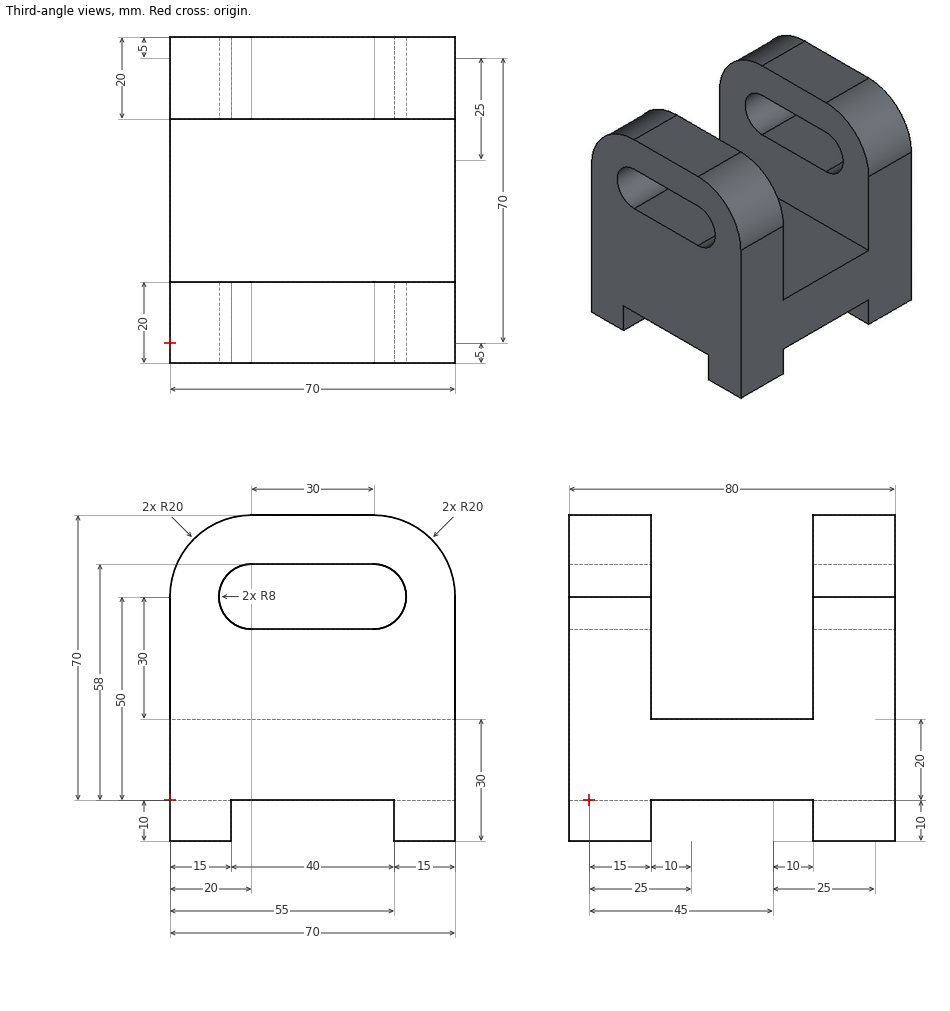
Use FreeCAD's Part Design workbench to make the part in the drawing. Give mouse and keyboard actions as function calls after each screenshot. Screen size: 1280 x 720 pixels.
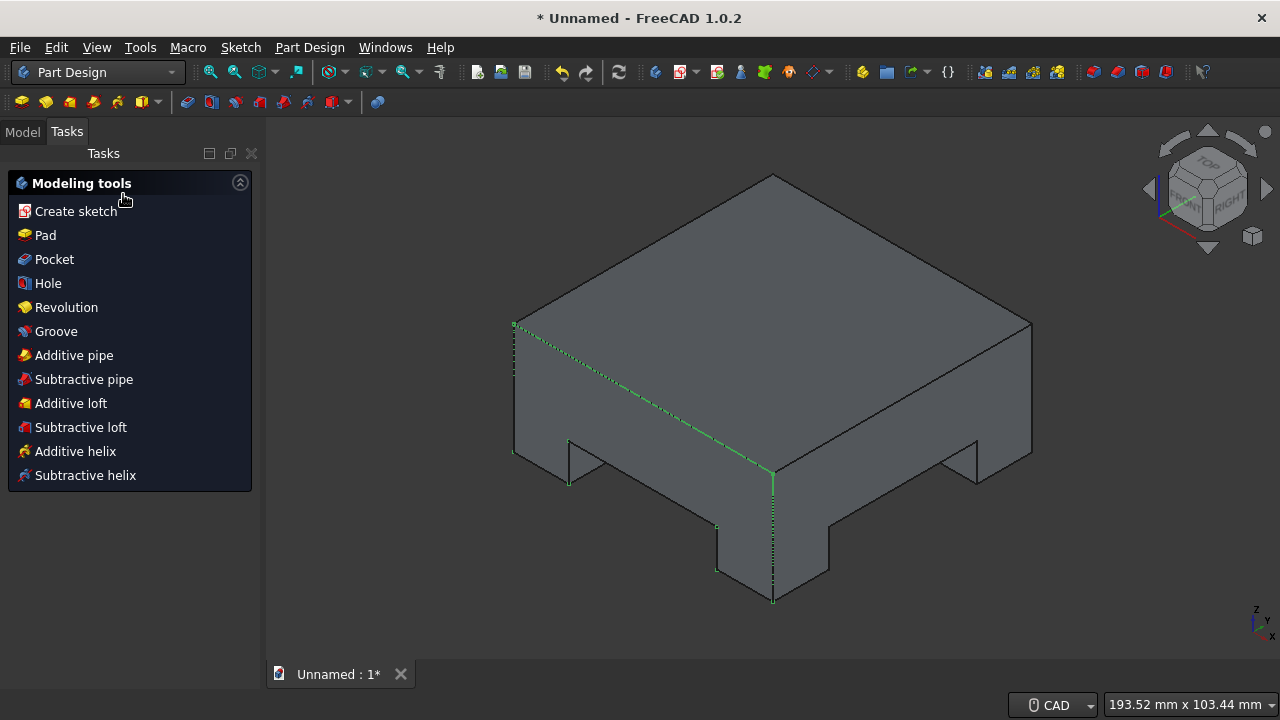
click(22, 102)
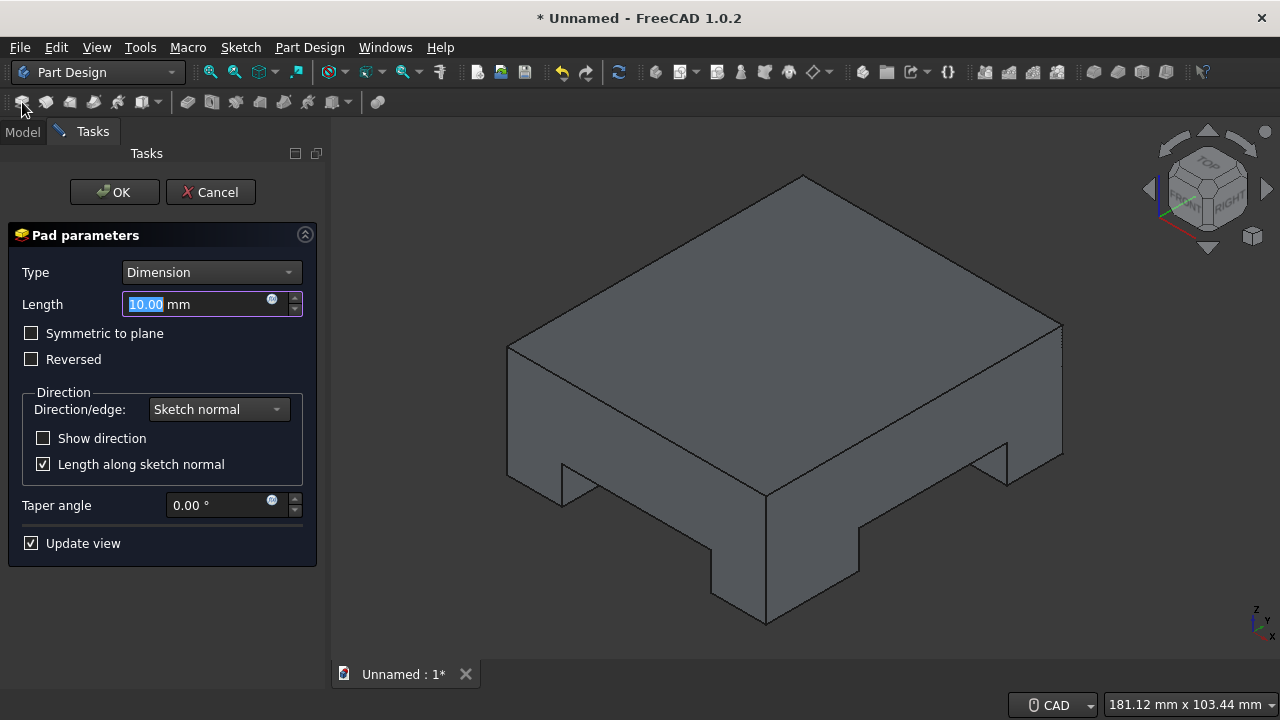
text(5)
key(Tab)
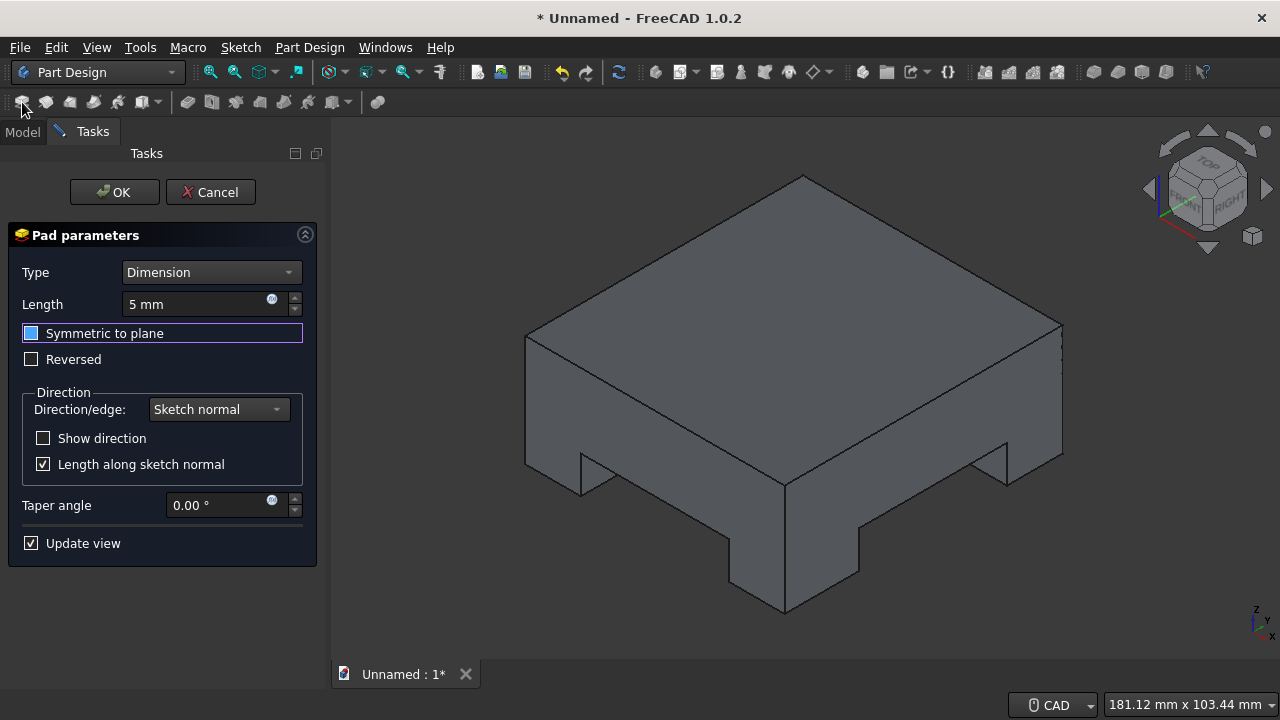
click(115, 192)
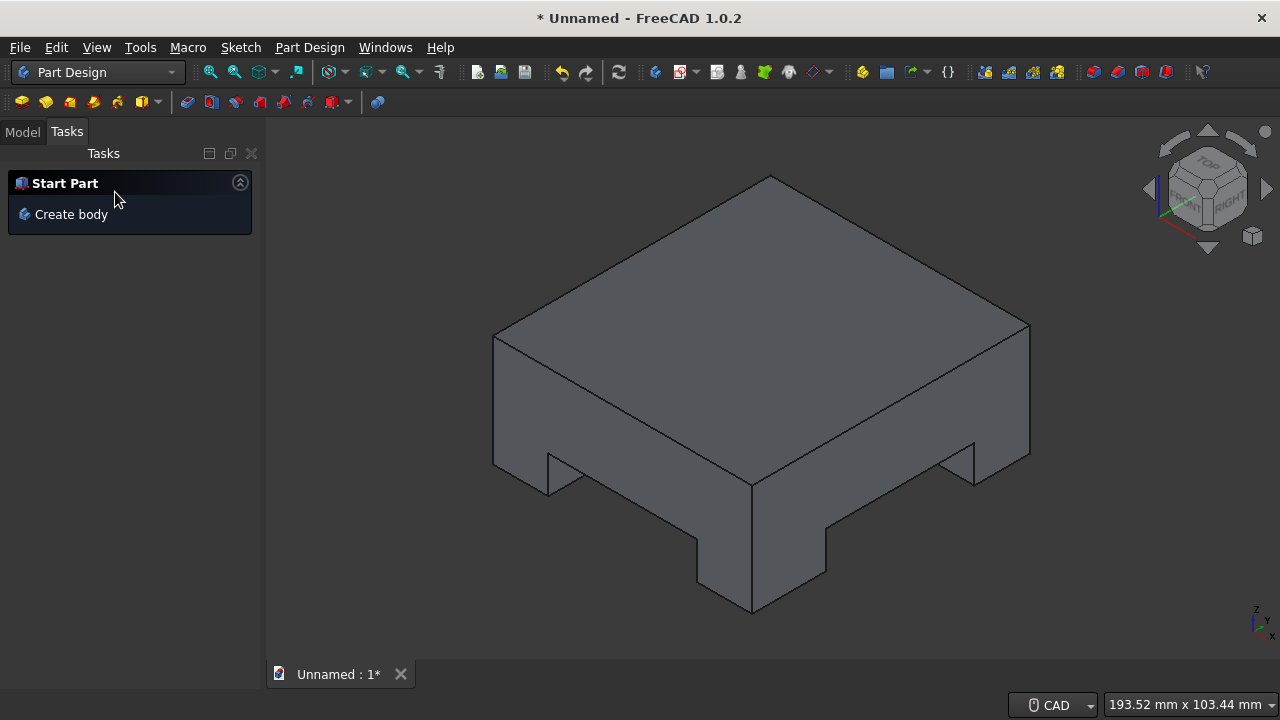
key(4)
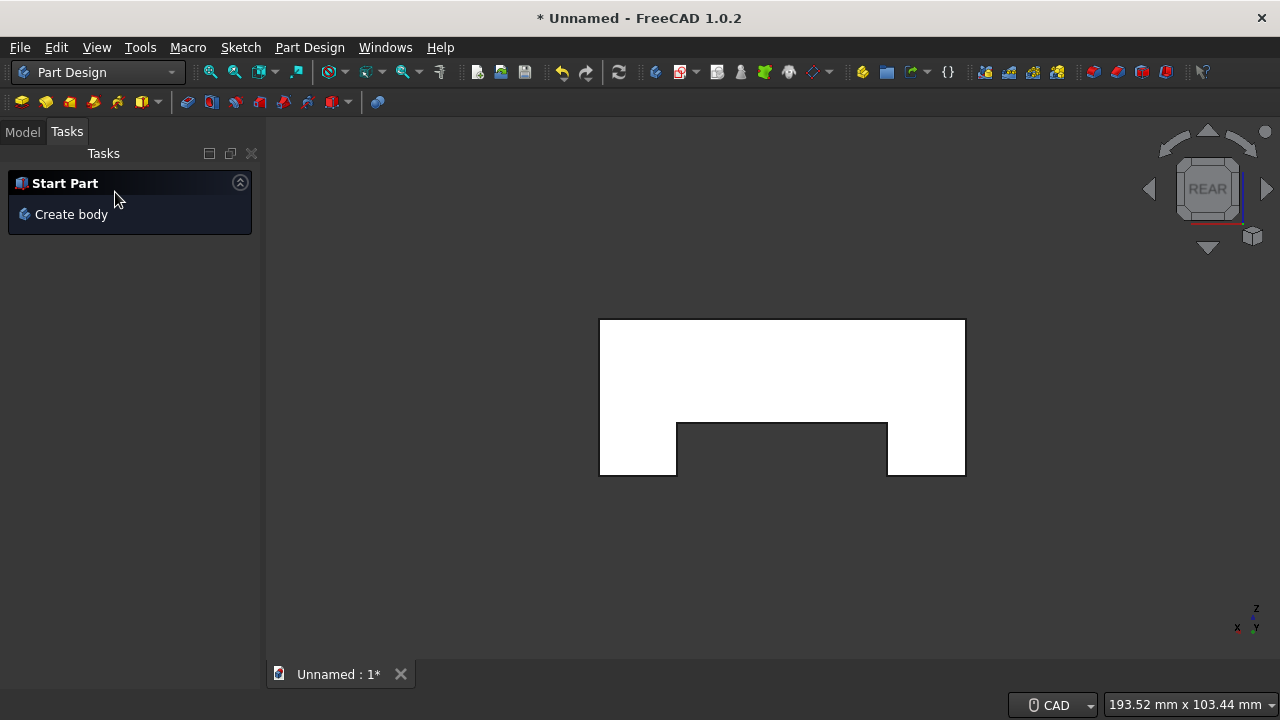
key(v)
key(f)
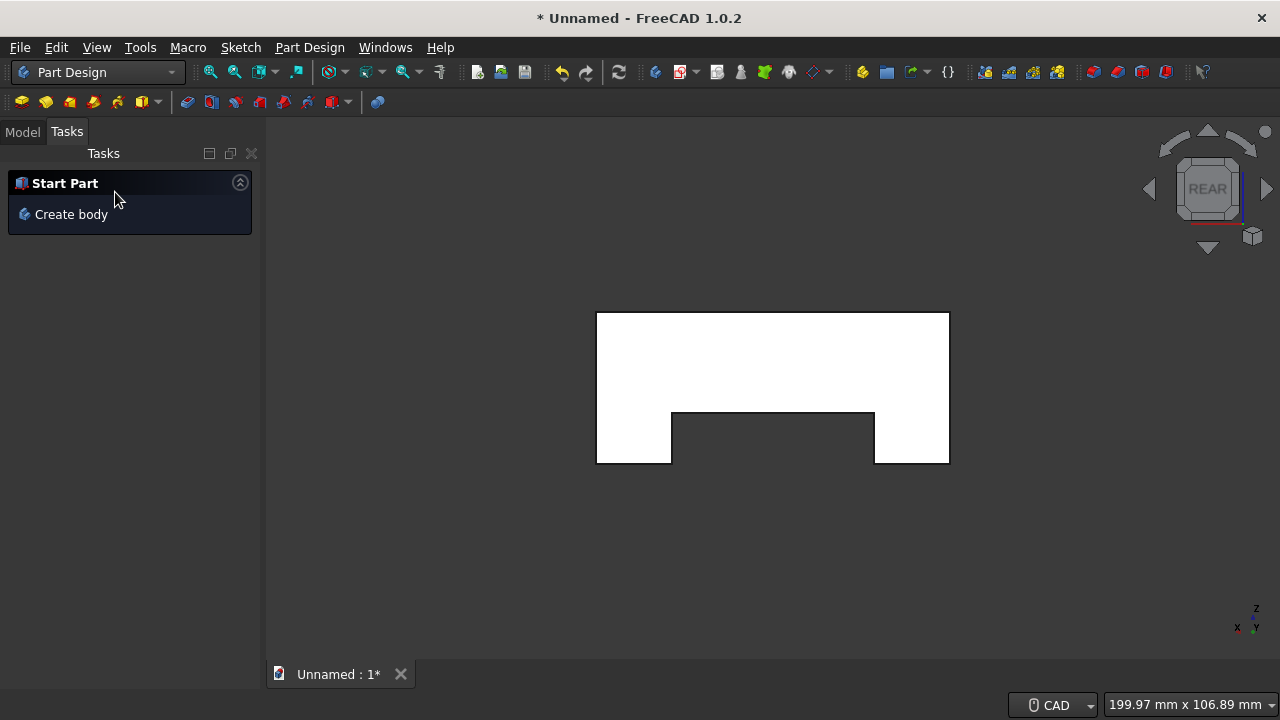
click(672, 365)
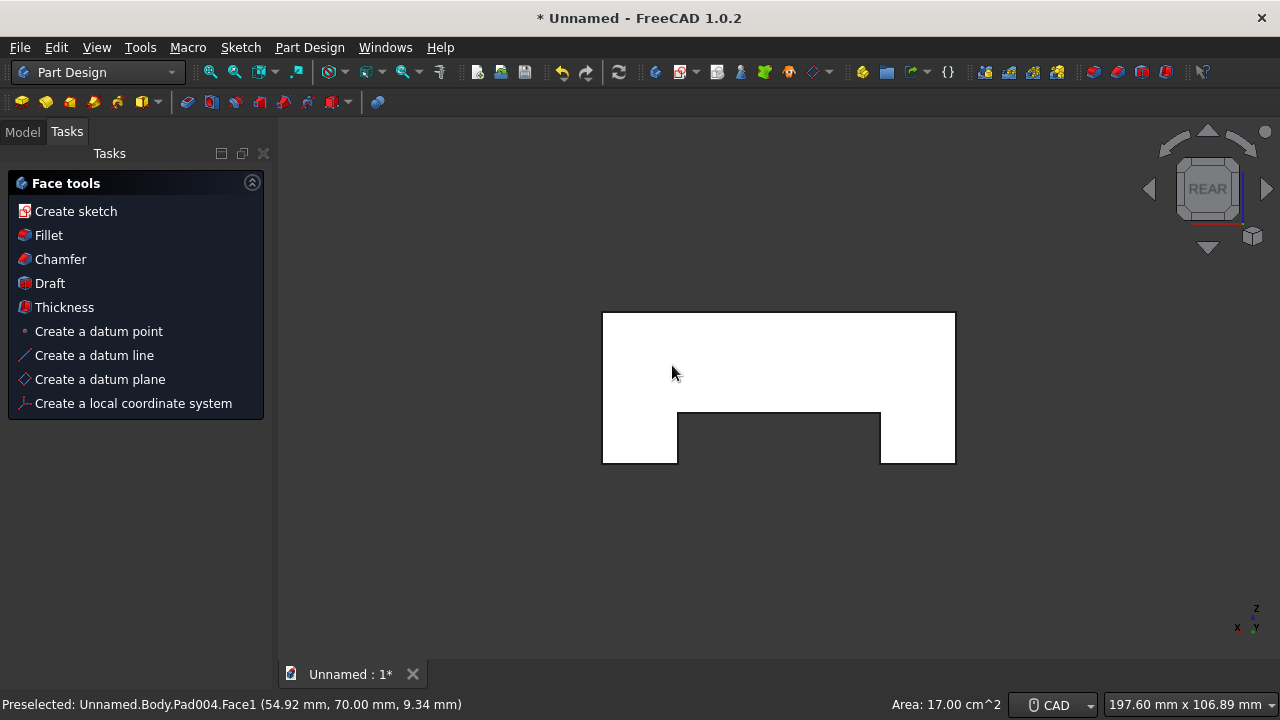
click(680, 72)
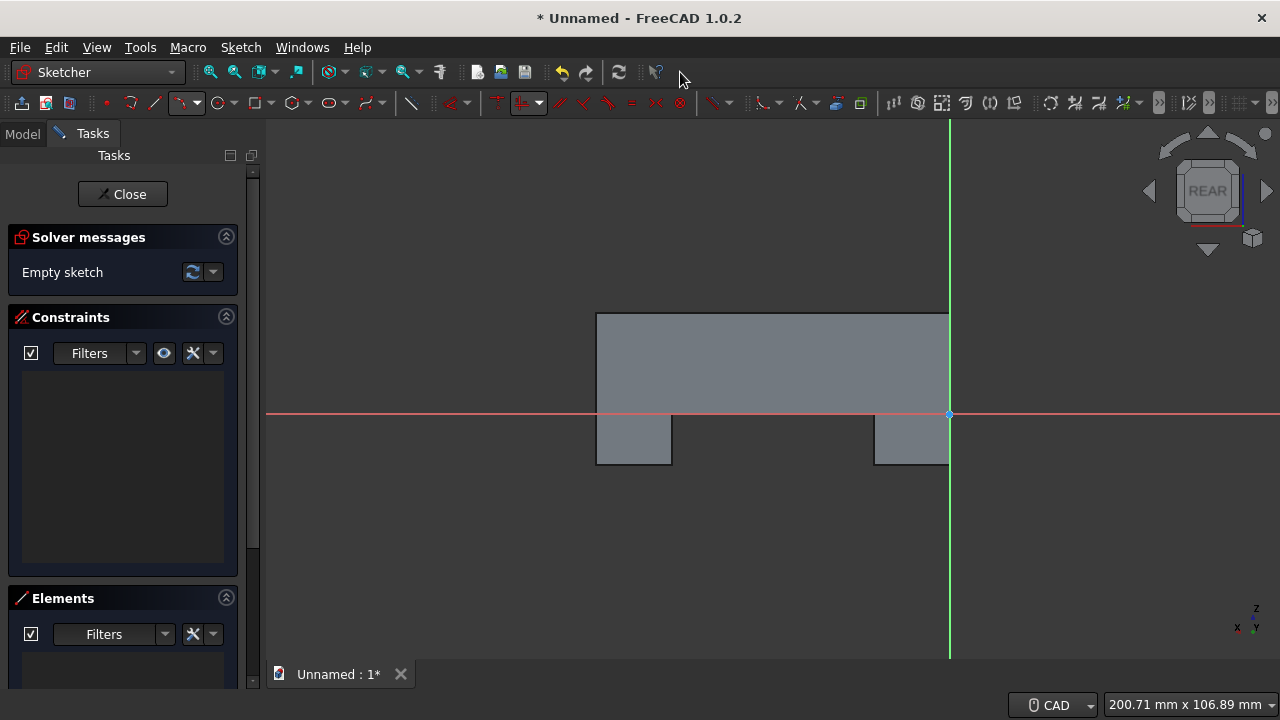
scroll(912, 389, up, 2)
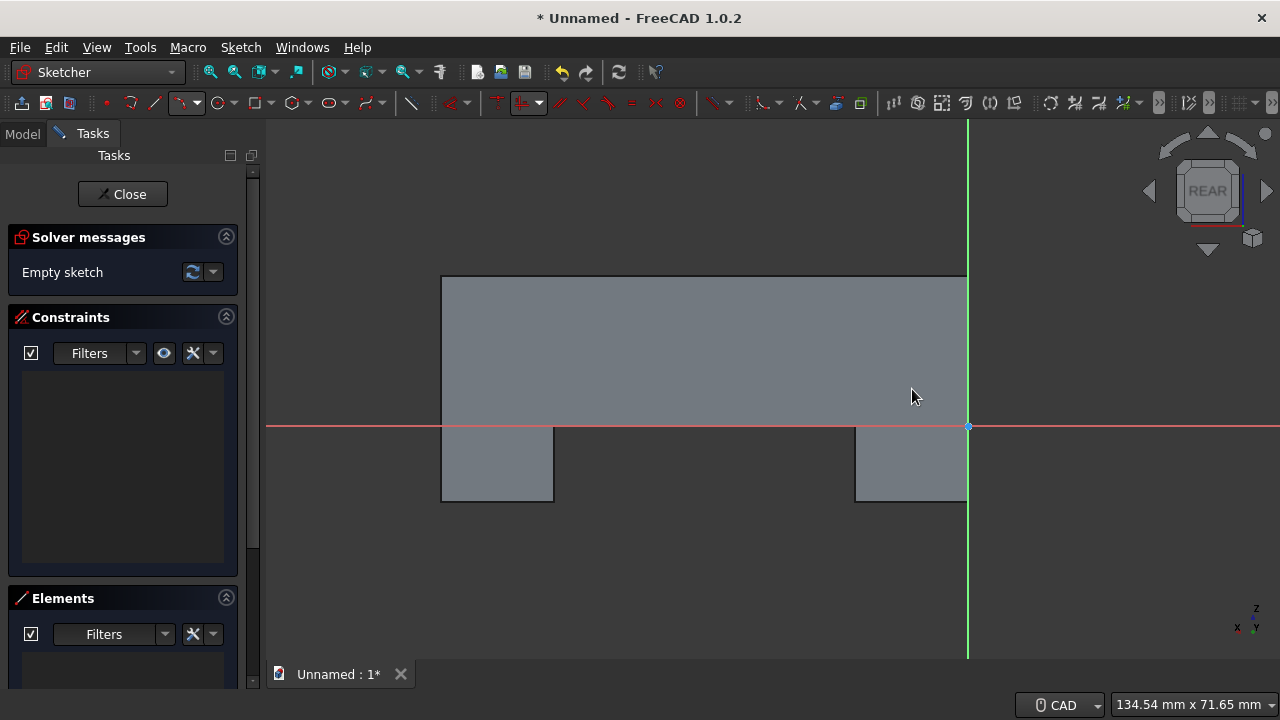
key(g)
key(m)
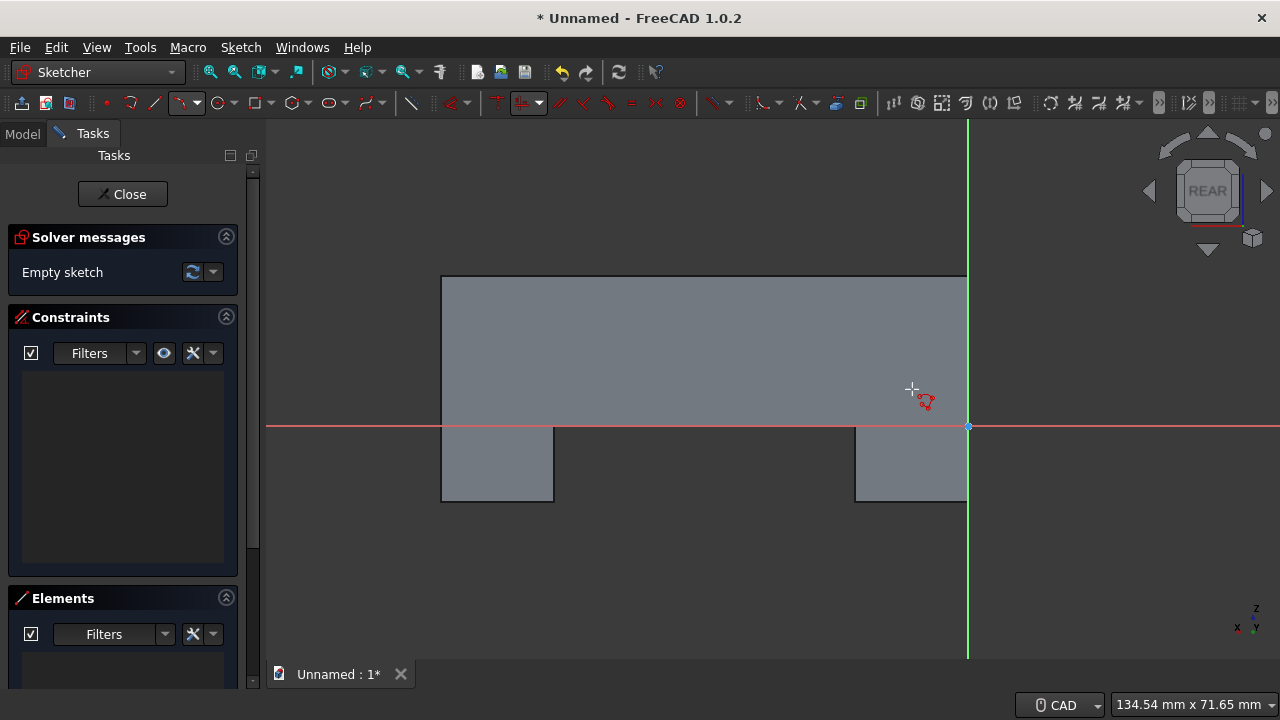
click(968, 502)
click(959, 276)
click(441, 276)
click(441, 502)
click(554, 502)
click(554, 426)
click(855, 417)
click(855, 502)
click(968, 503)
key(Escape)
key(Escape)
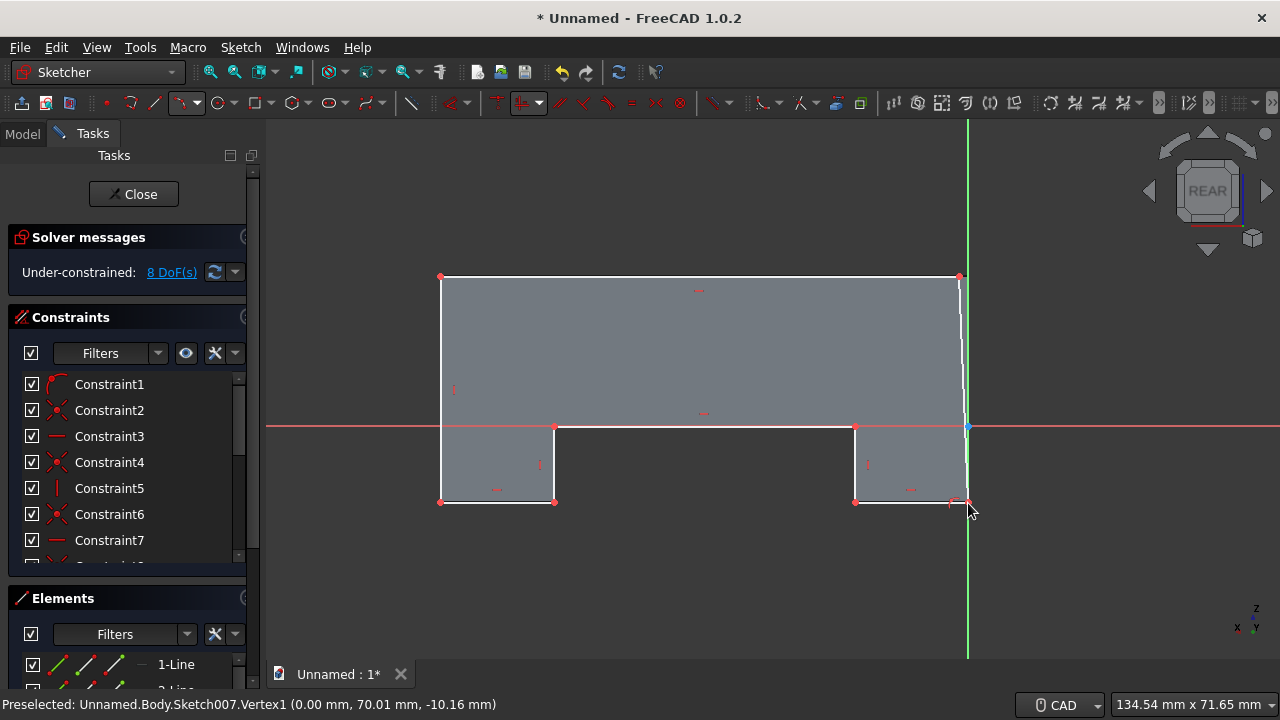
click(964, 413)